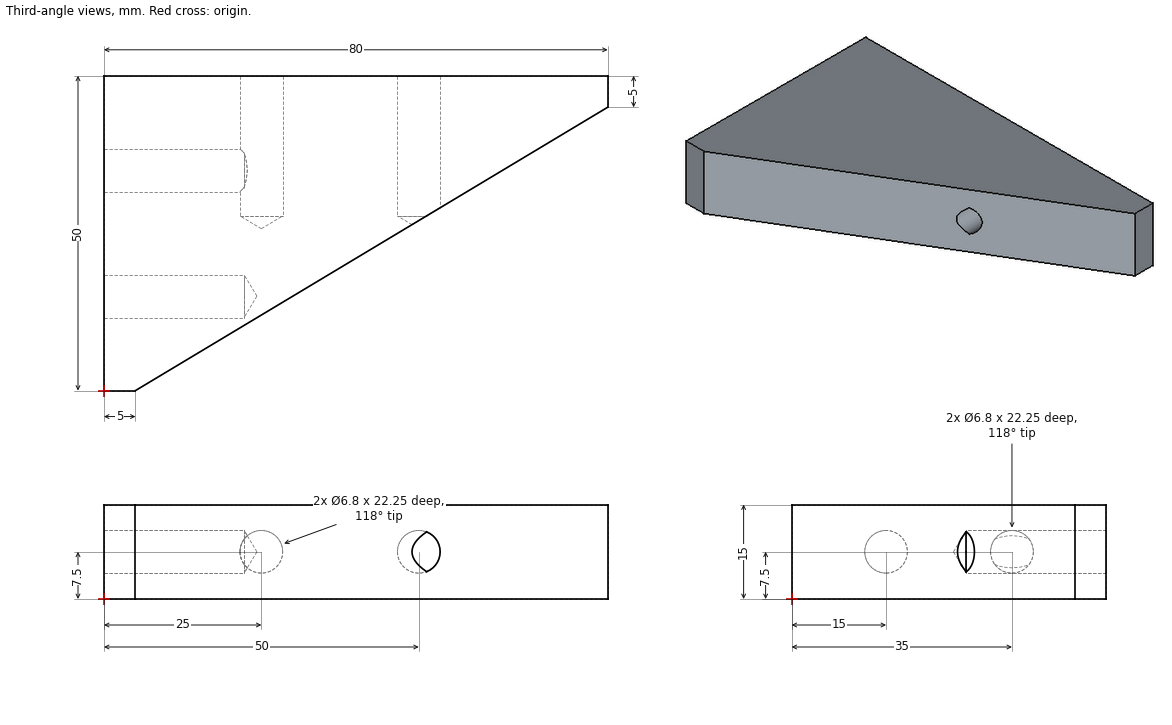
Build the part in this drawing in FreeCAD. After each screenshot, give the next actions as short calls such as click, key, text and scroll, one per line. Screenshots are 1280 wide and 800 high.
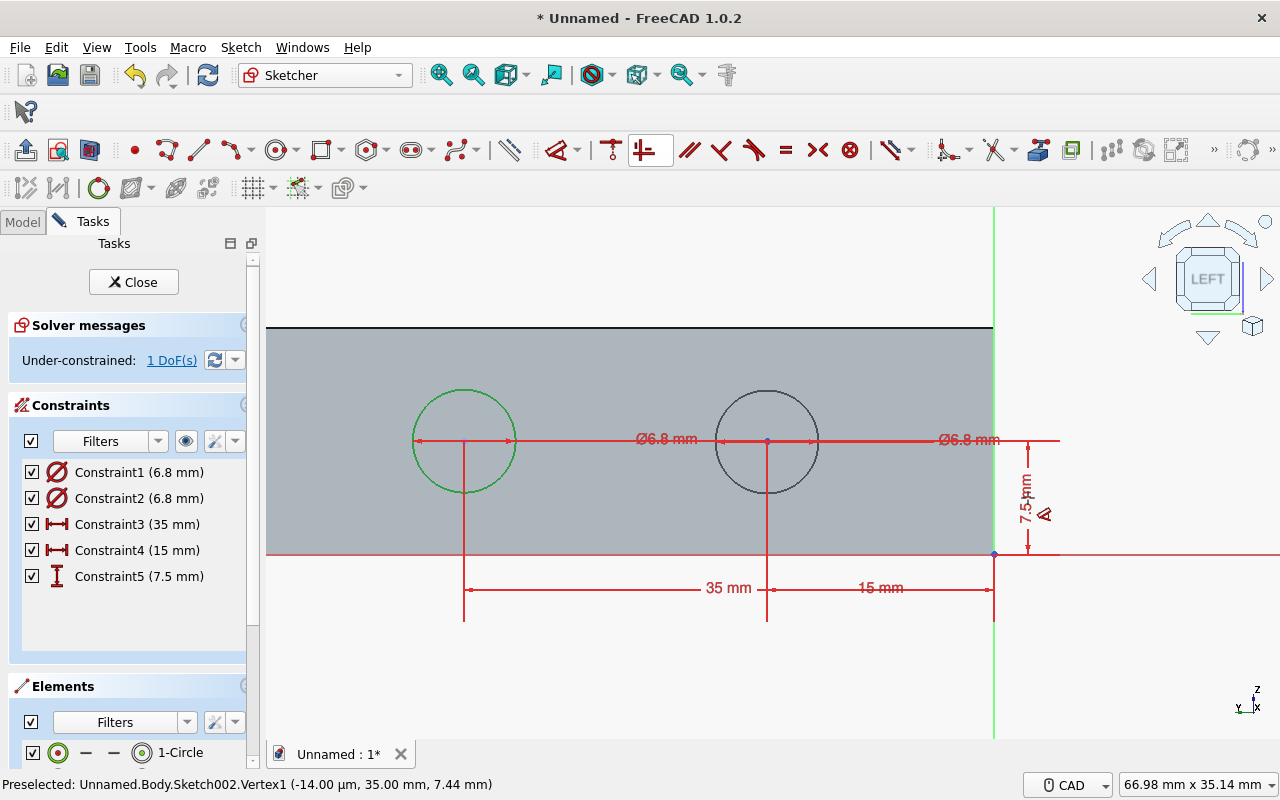
click(767, 442)
click(1028, 472)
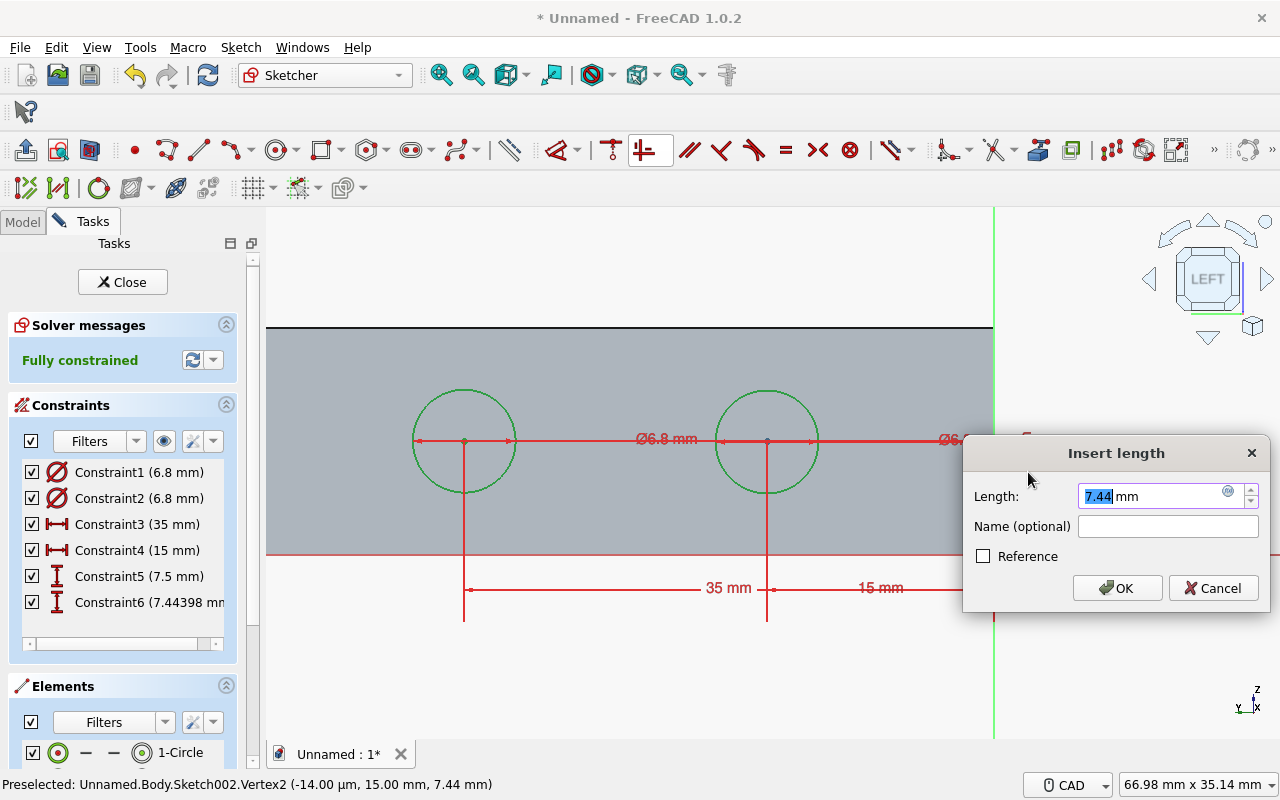
text(7.5)
key(Return)
key(Escape)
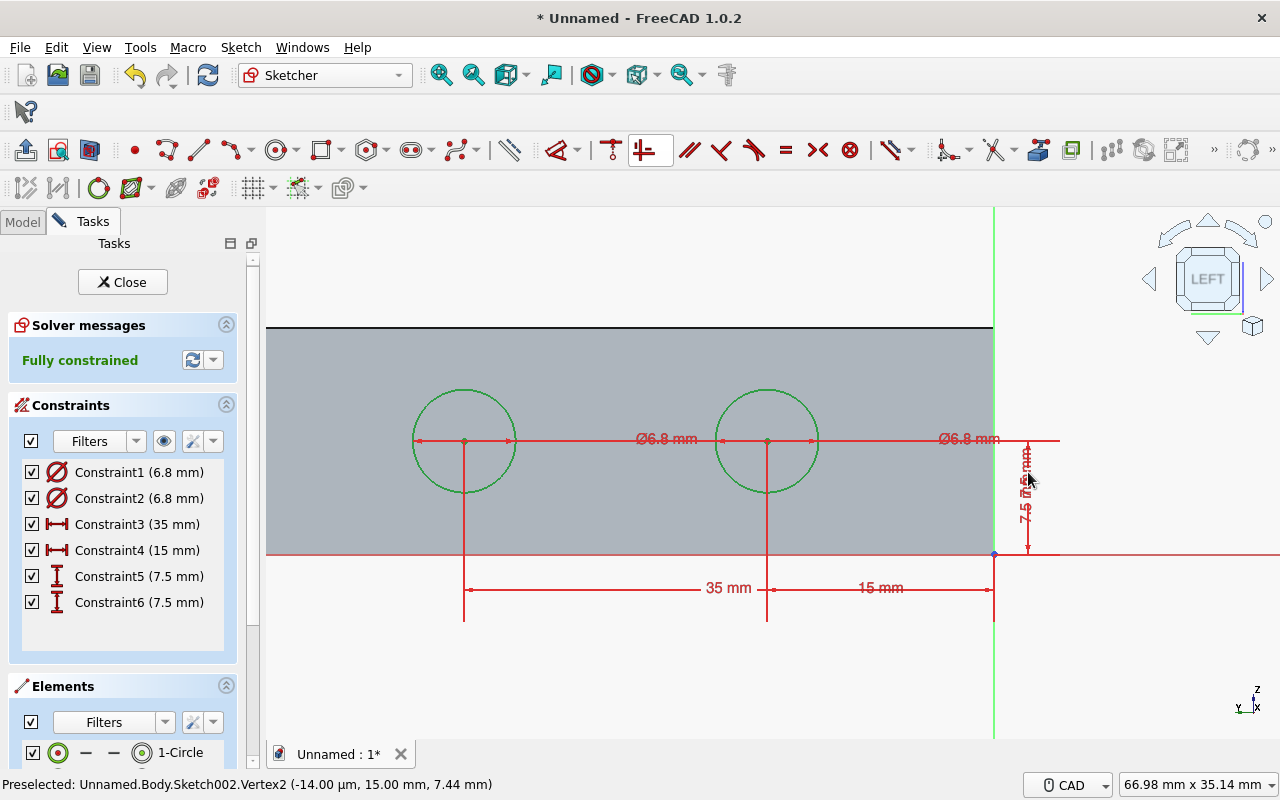
click(123, 282)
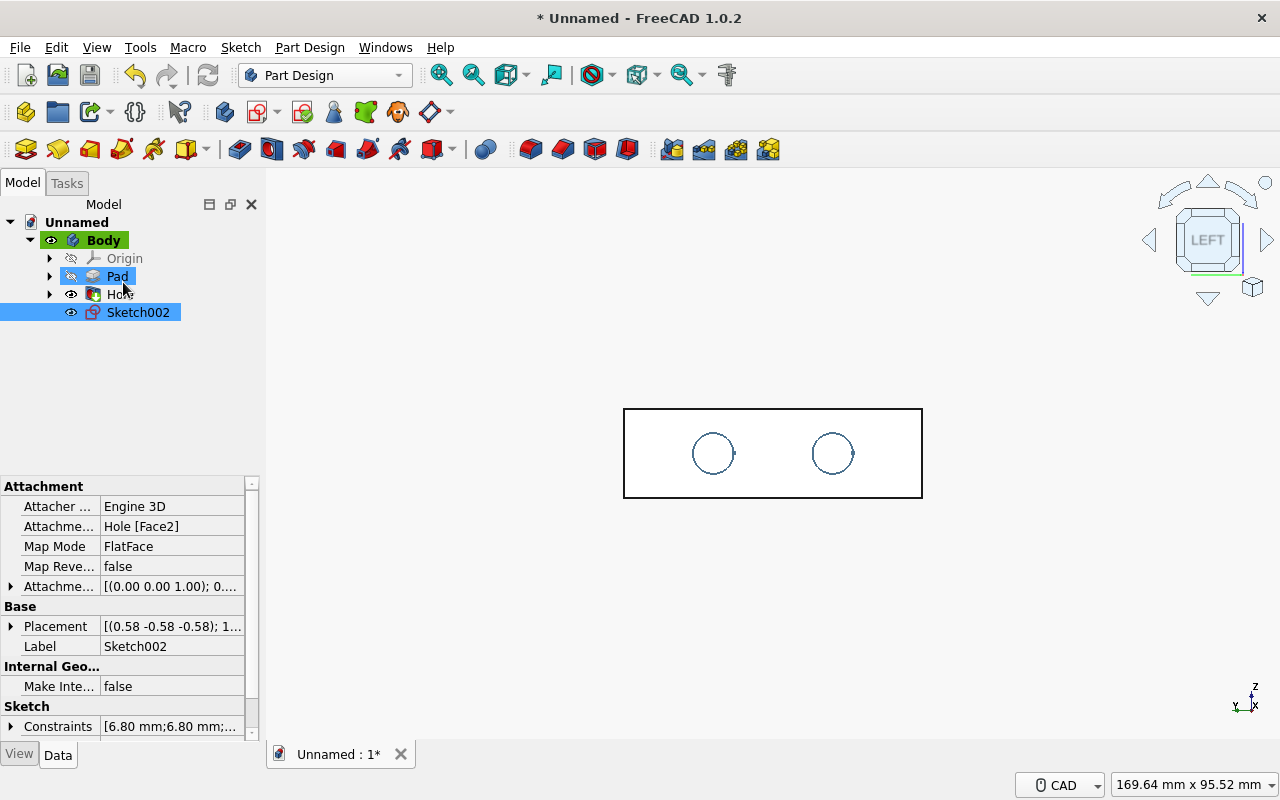
click(272, 150)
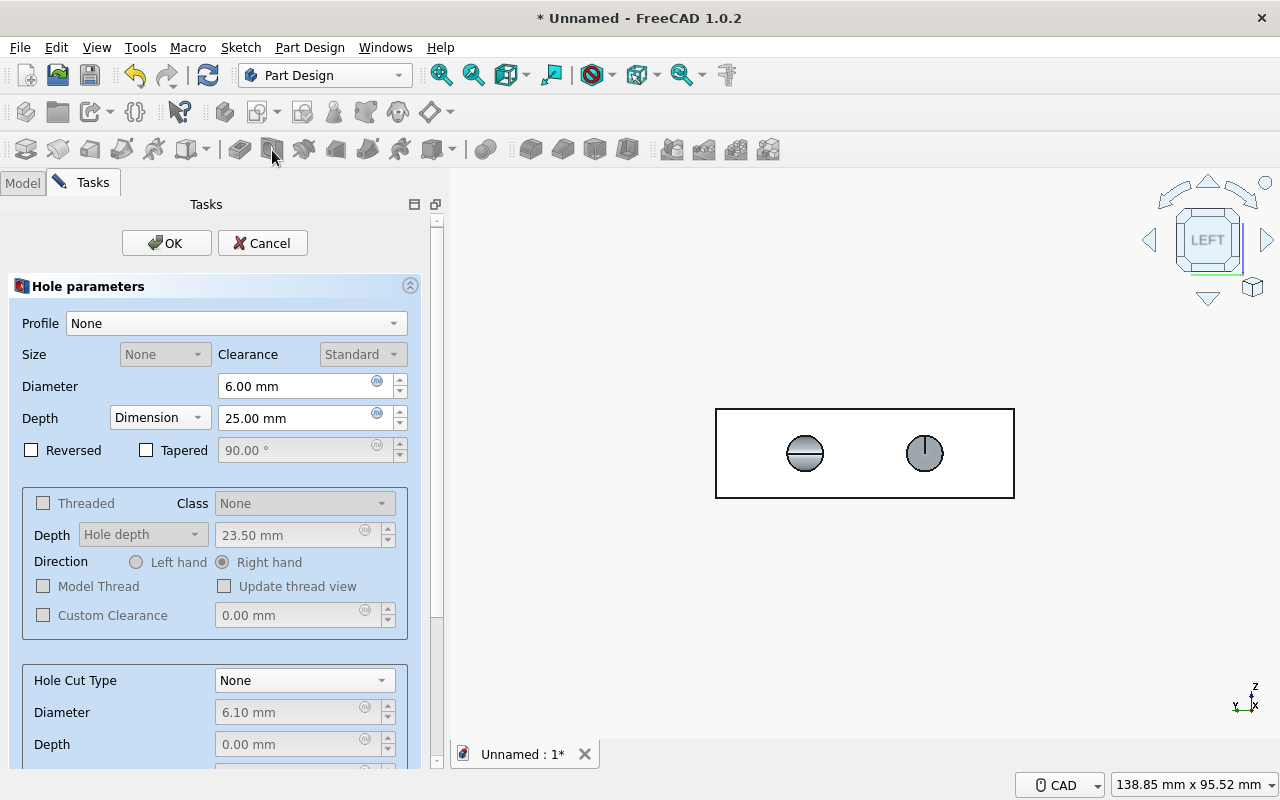
triple_click(305, 386)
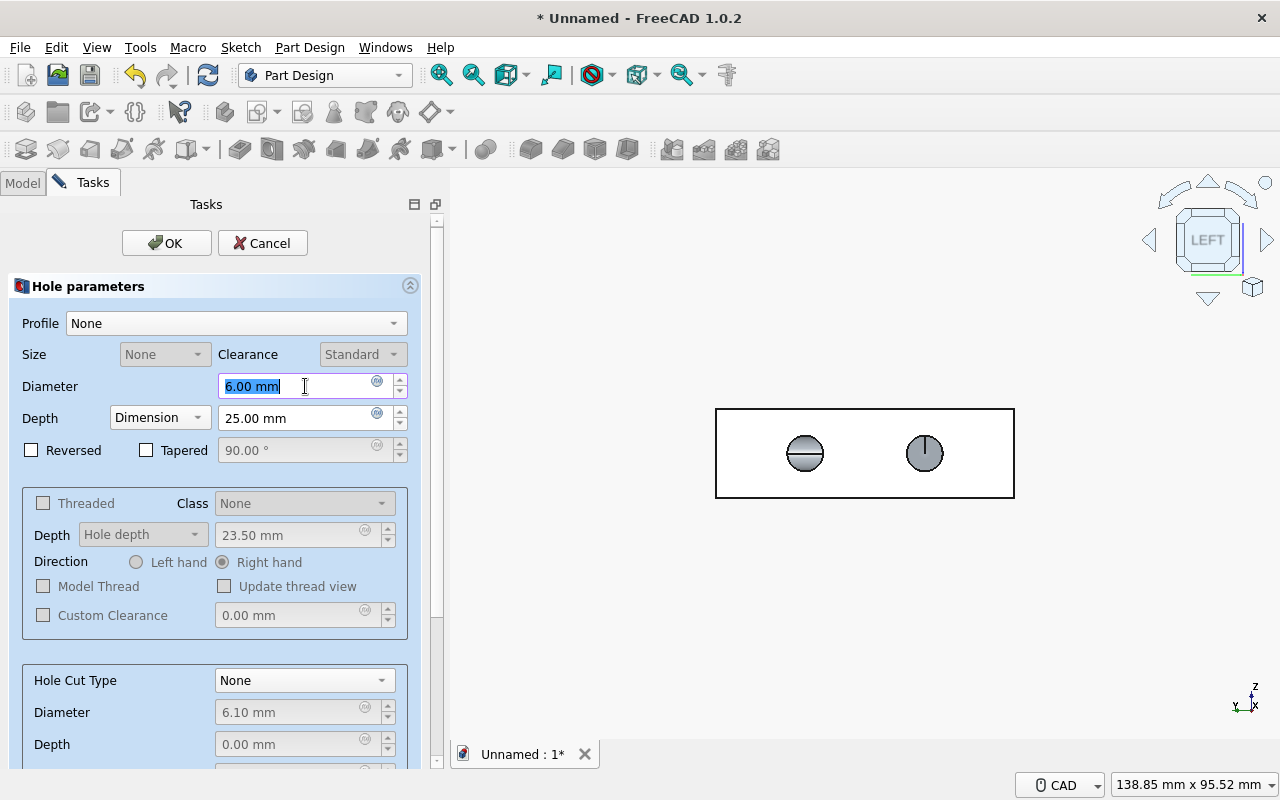
text(6.8)
key(Tab)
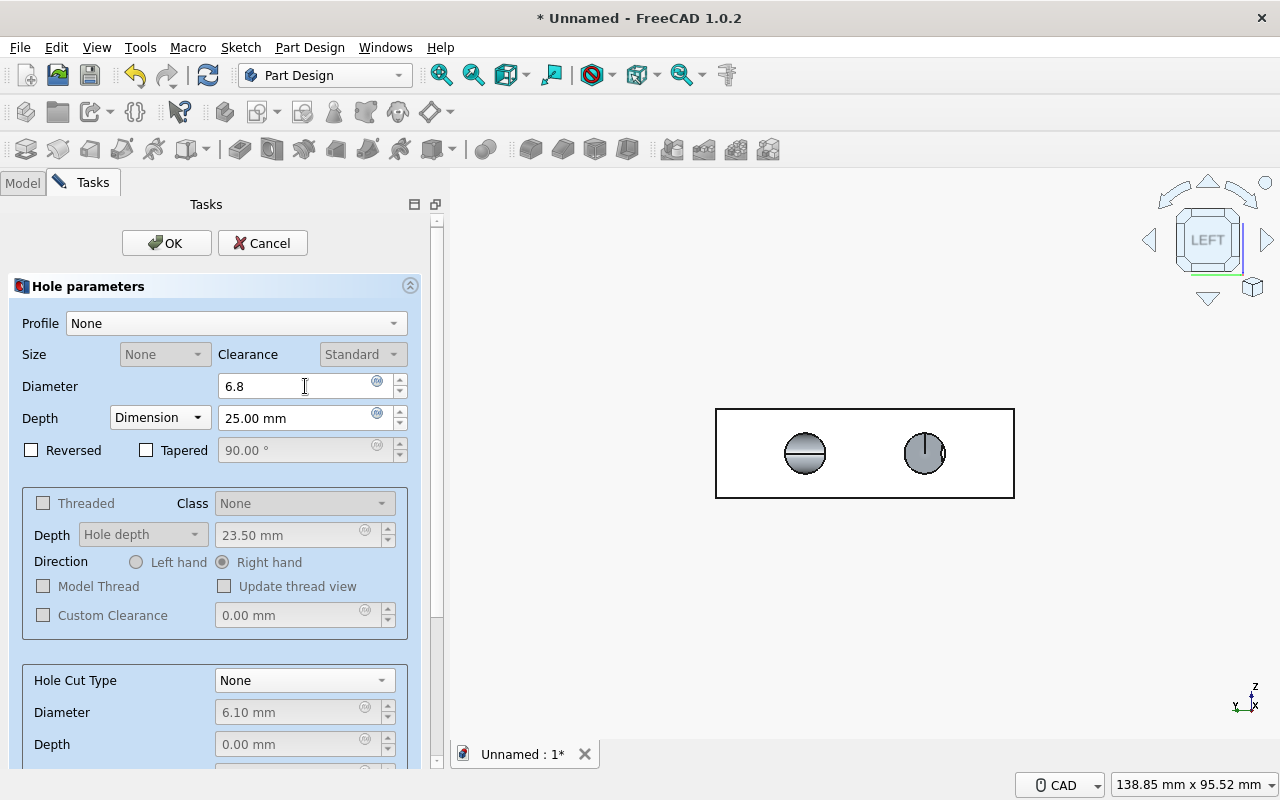
triple_click(305, 418)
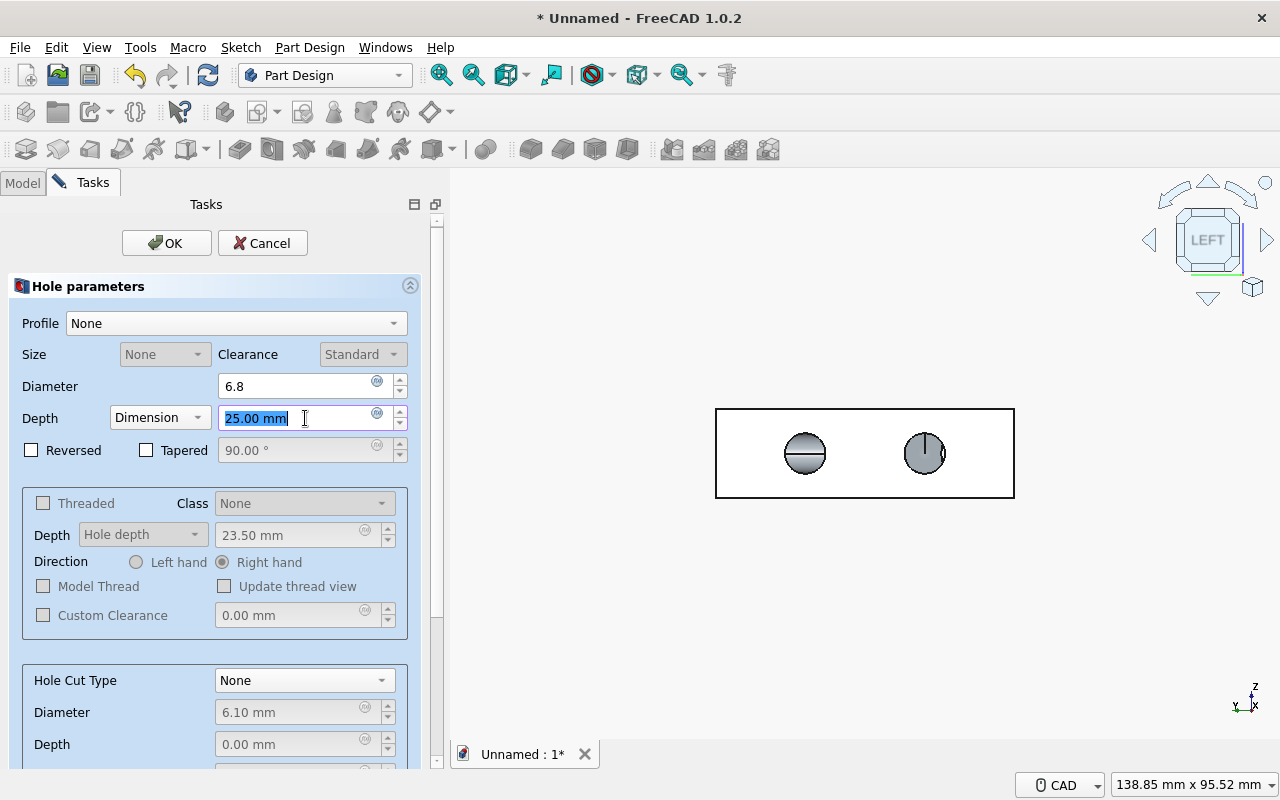
text(22.25)
key(Tab)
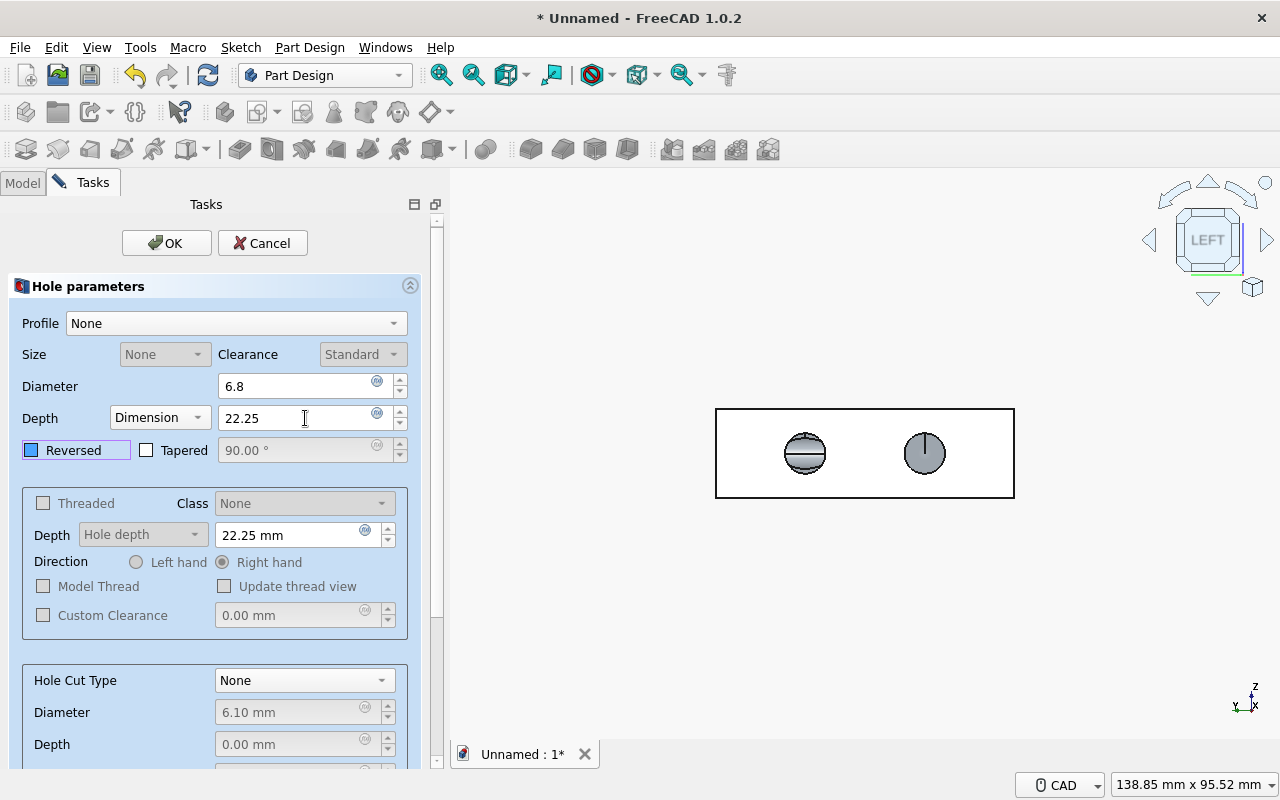
click(167, 243)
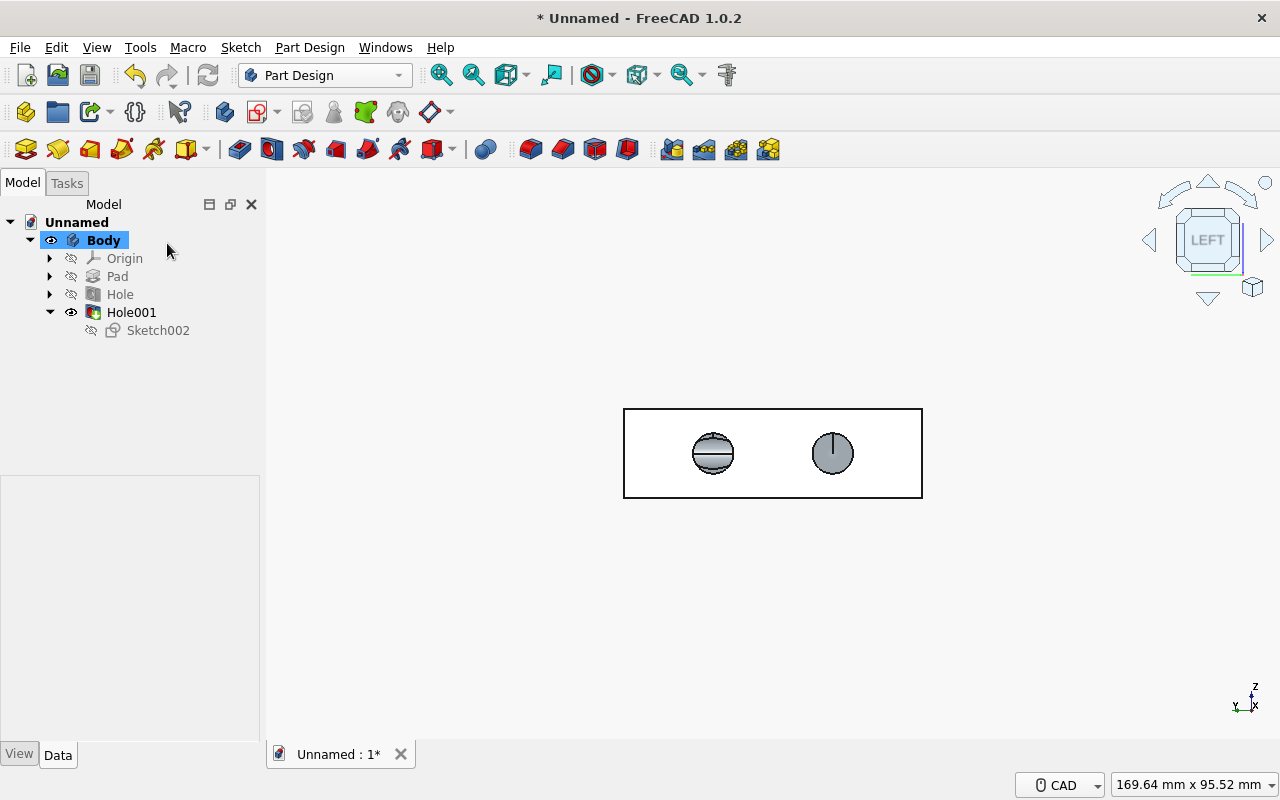
key(0)